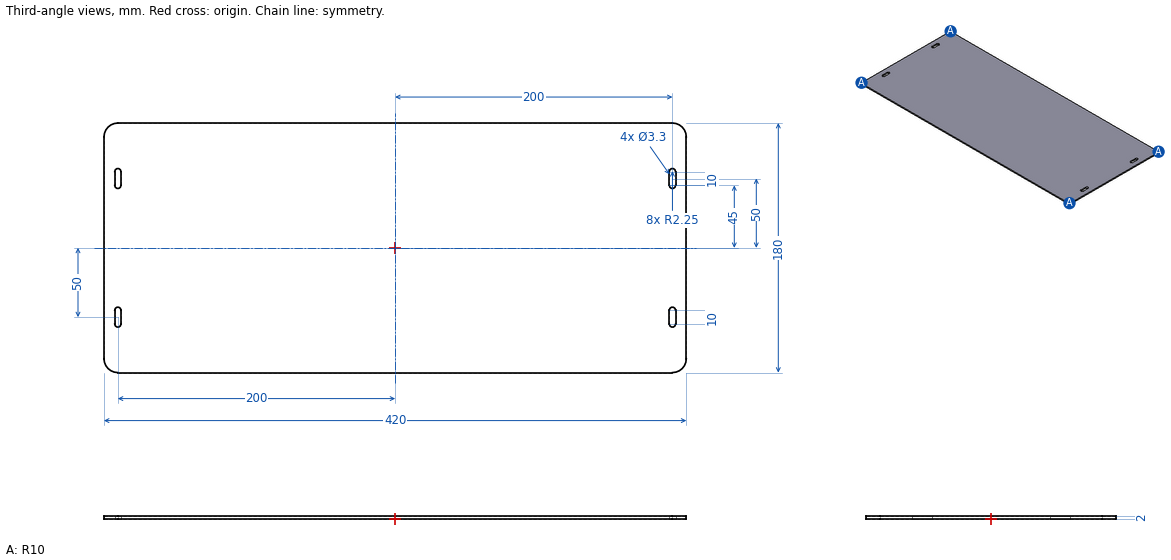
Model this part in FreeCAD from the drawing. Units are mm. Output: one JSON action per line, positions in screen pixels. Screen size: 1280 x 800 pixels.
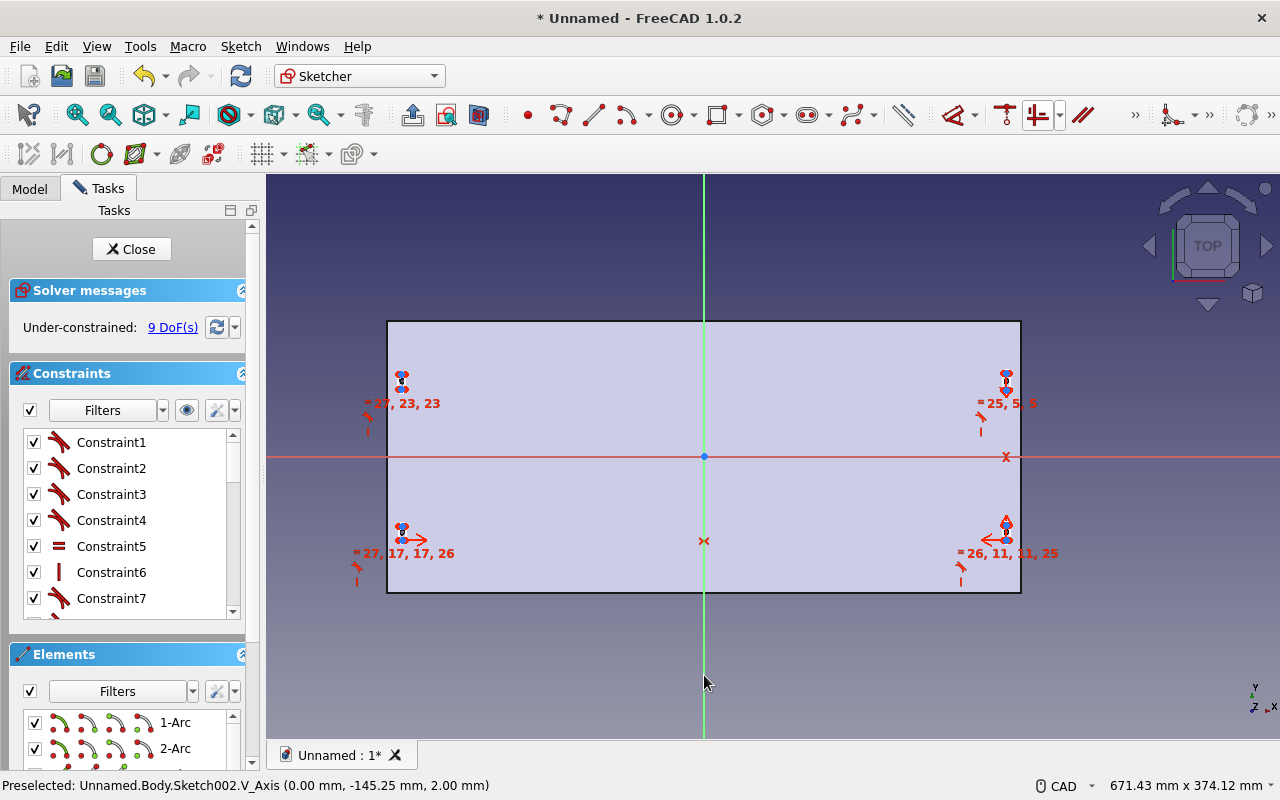
{"action": "scroll", "coordinate": [1006, 390], "scroll_direction": "up", "scroll_amount": 7}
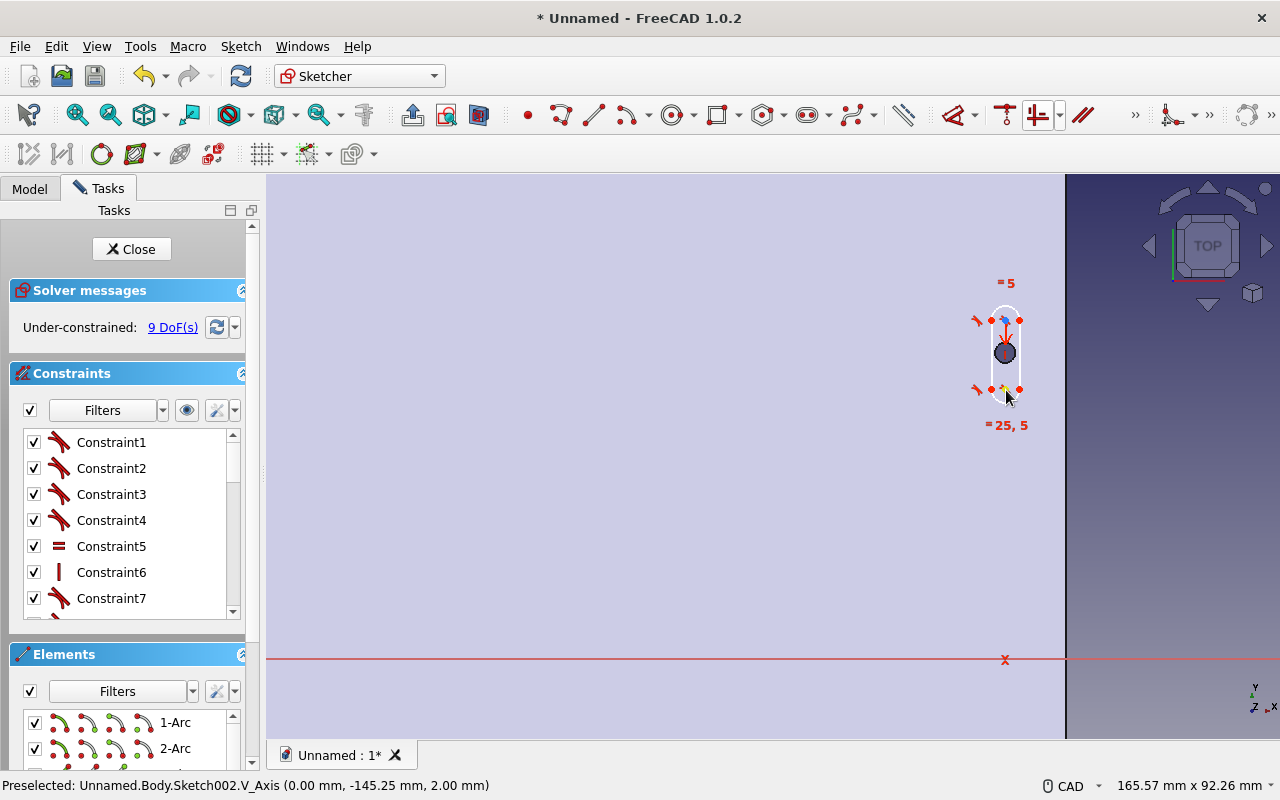
{"action": "left_click", "coordinate": [1006, 389]}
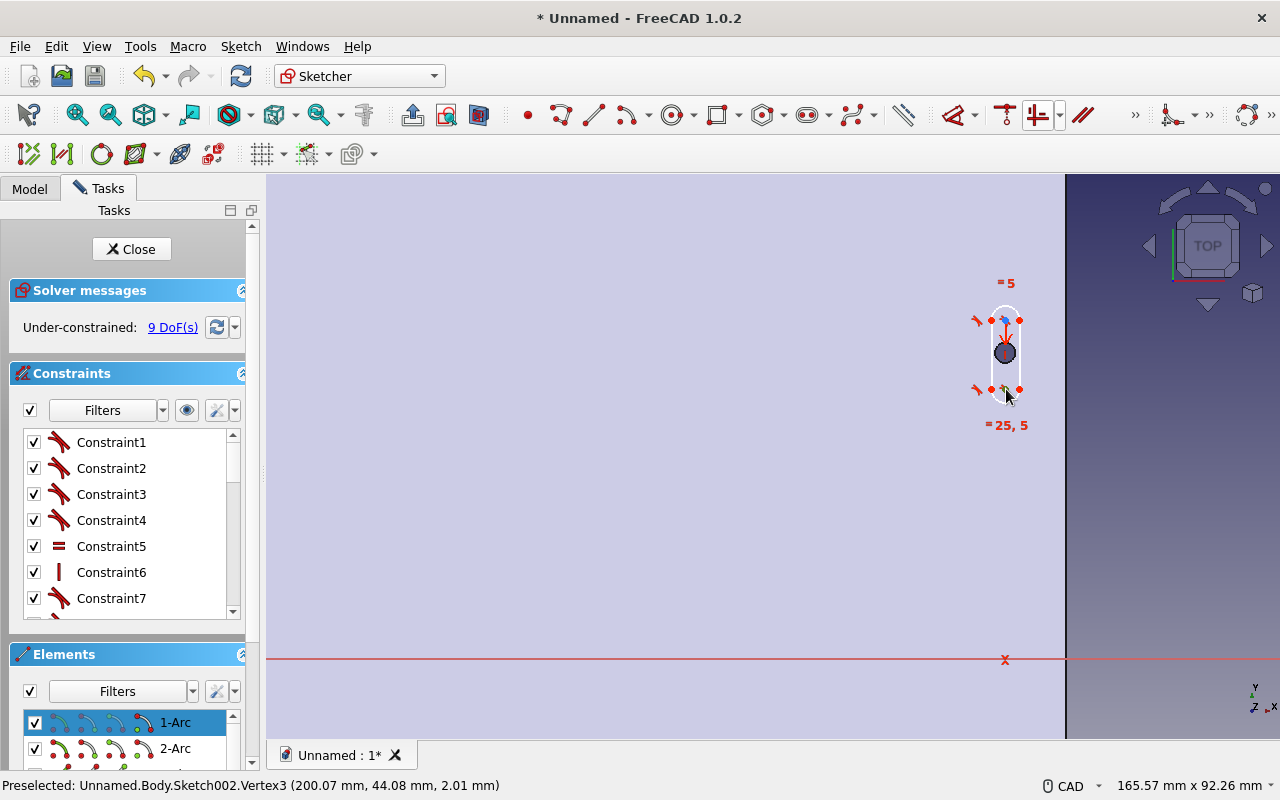
{"action": "scroll", "coordinate": [1007, 390], "scroll_direction": "down", "scroll_amount": 7}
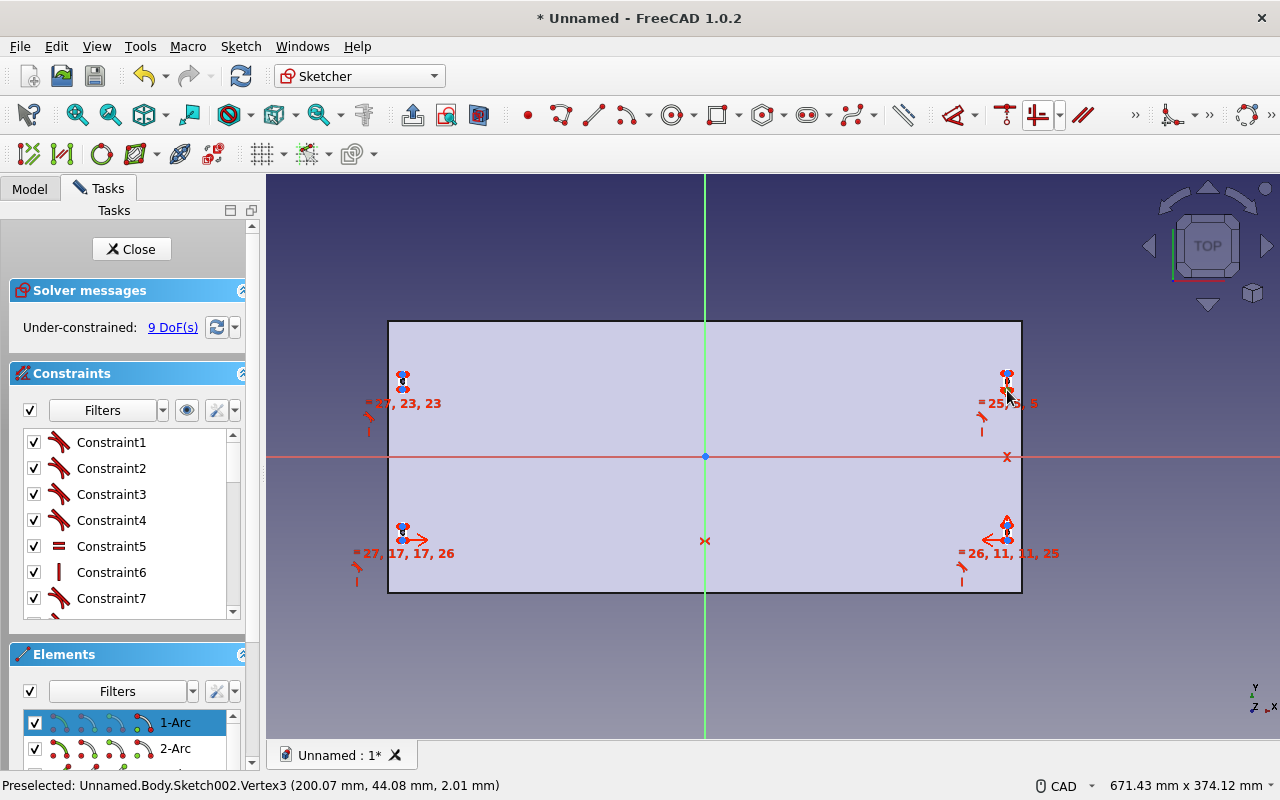
{"action": "scroll", "coordinate": [403, 390], "scroll_direction": "up", "scroll_amount": 7}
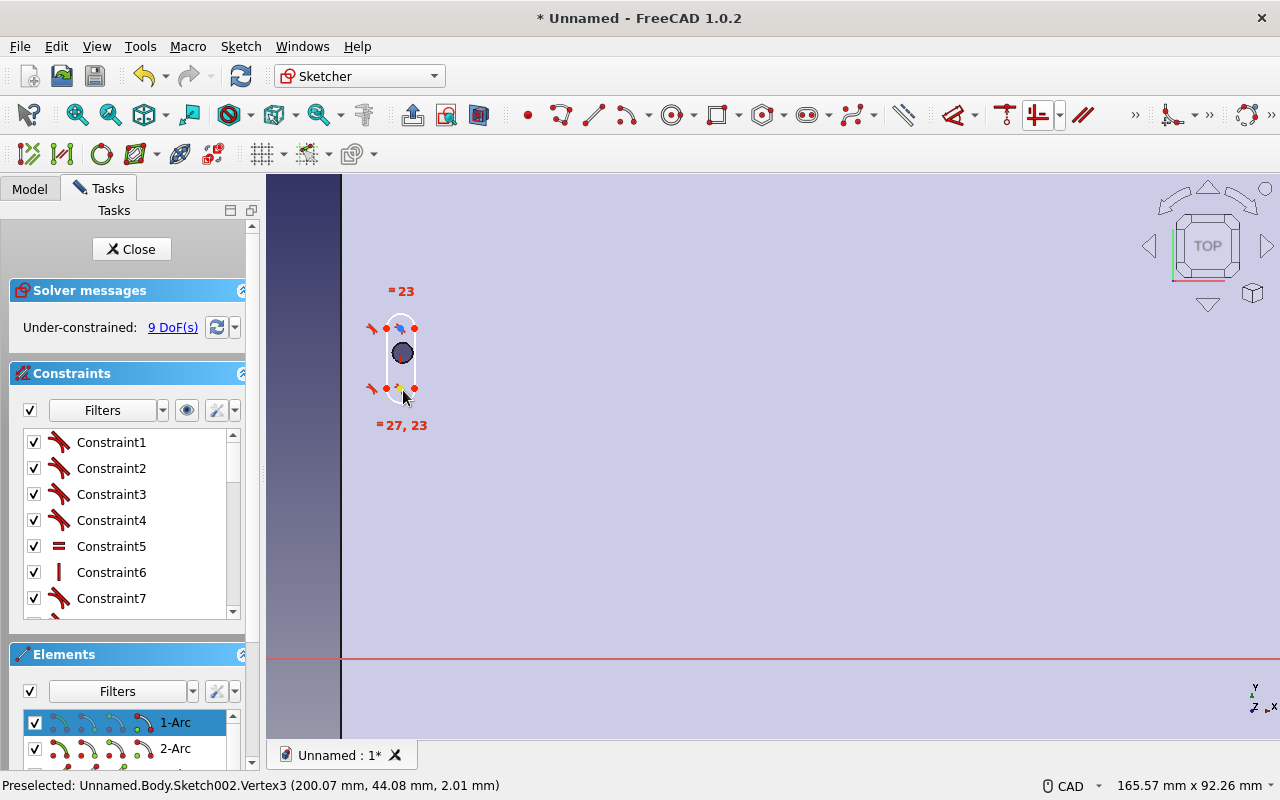
{"action": "left_click", "coordinate": [401, 389]}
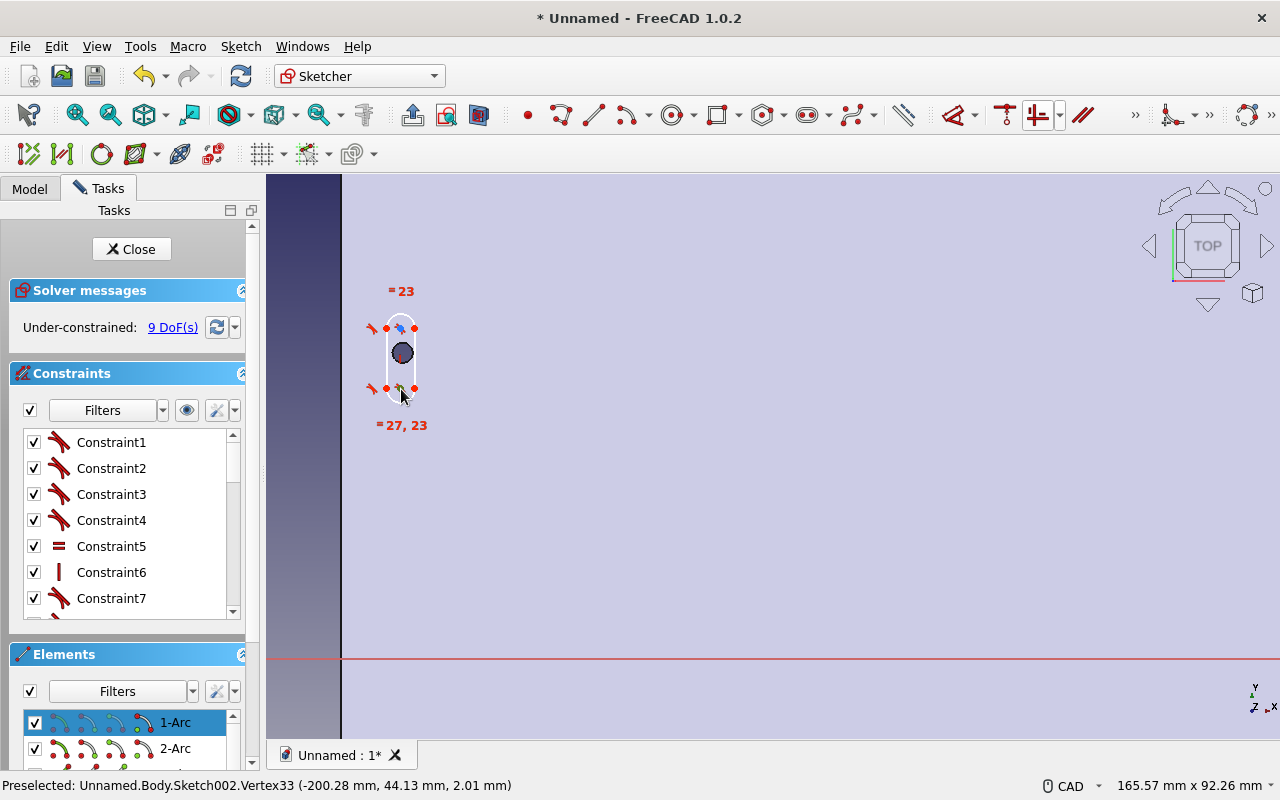
{"action": "scroll", "coordinate": [402, 390], "scroll_direction": "down", "scroll_amount": 7}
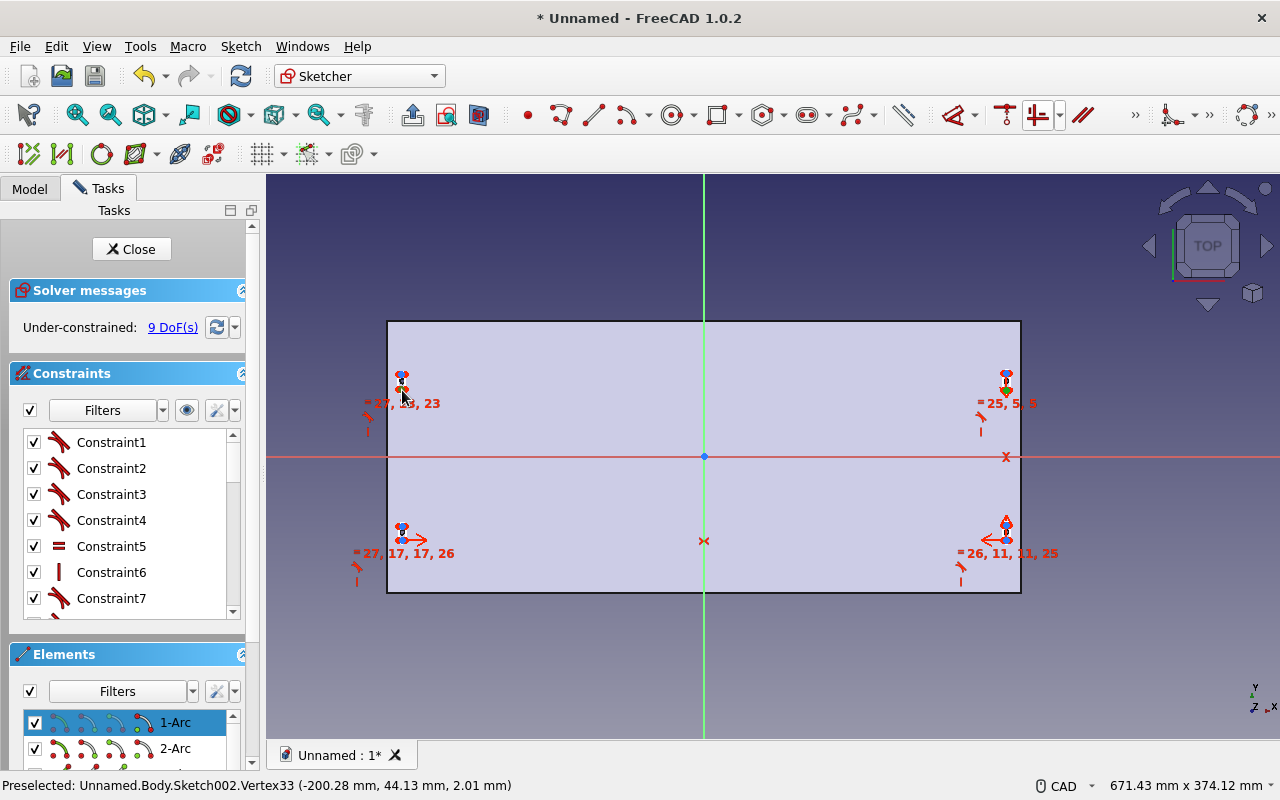
{"action": "left_click", "coordinate": [704, 675]}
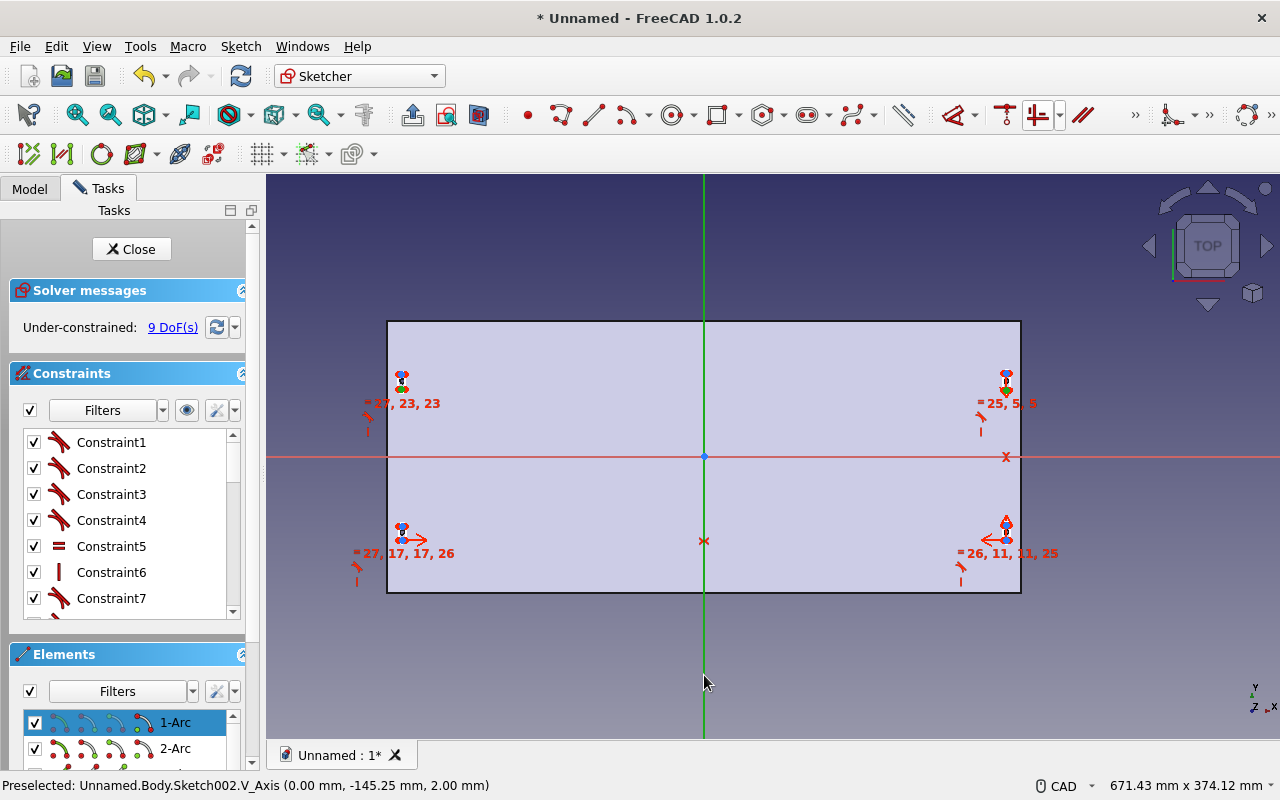
{"action": "key", "text": "s"}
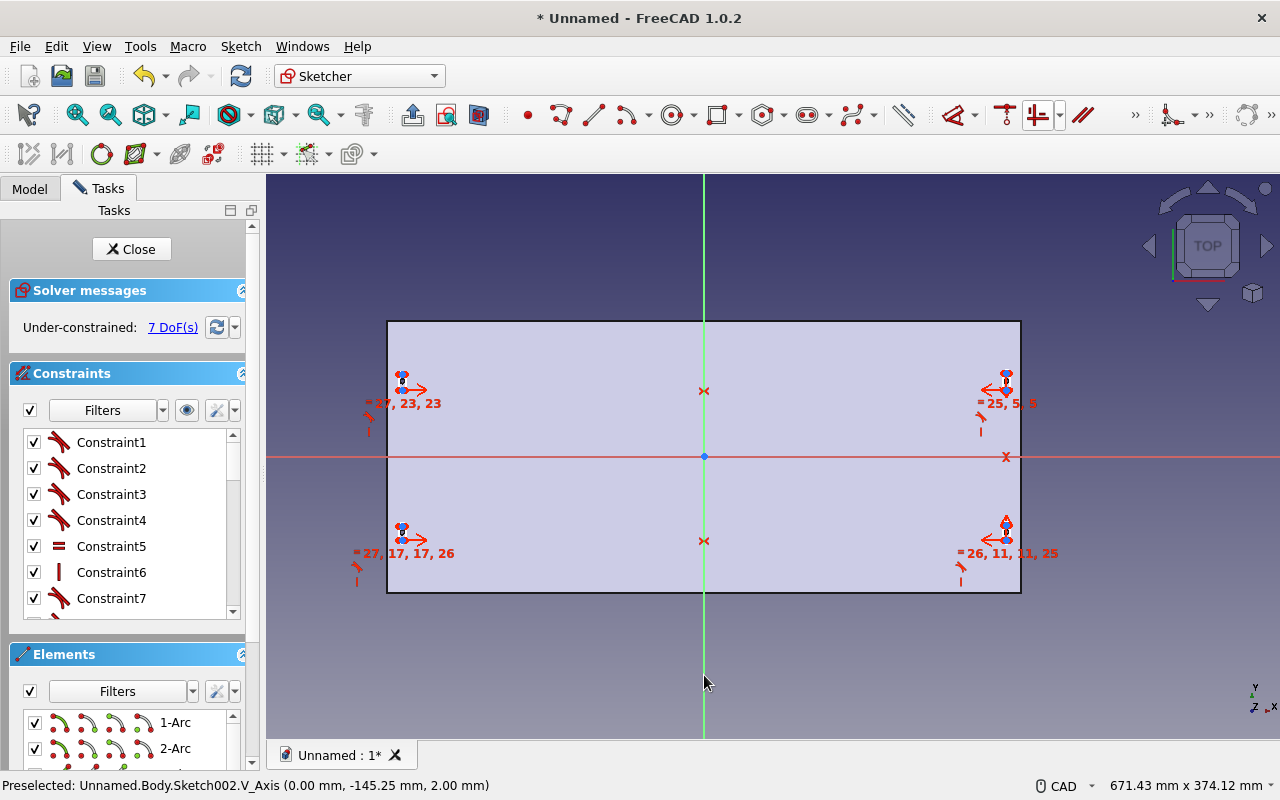
{"action": "key", "text": "d"}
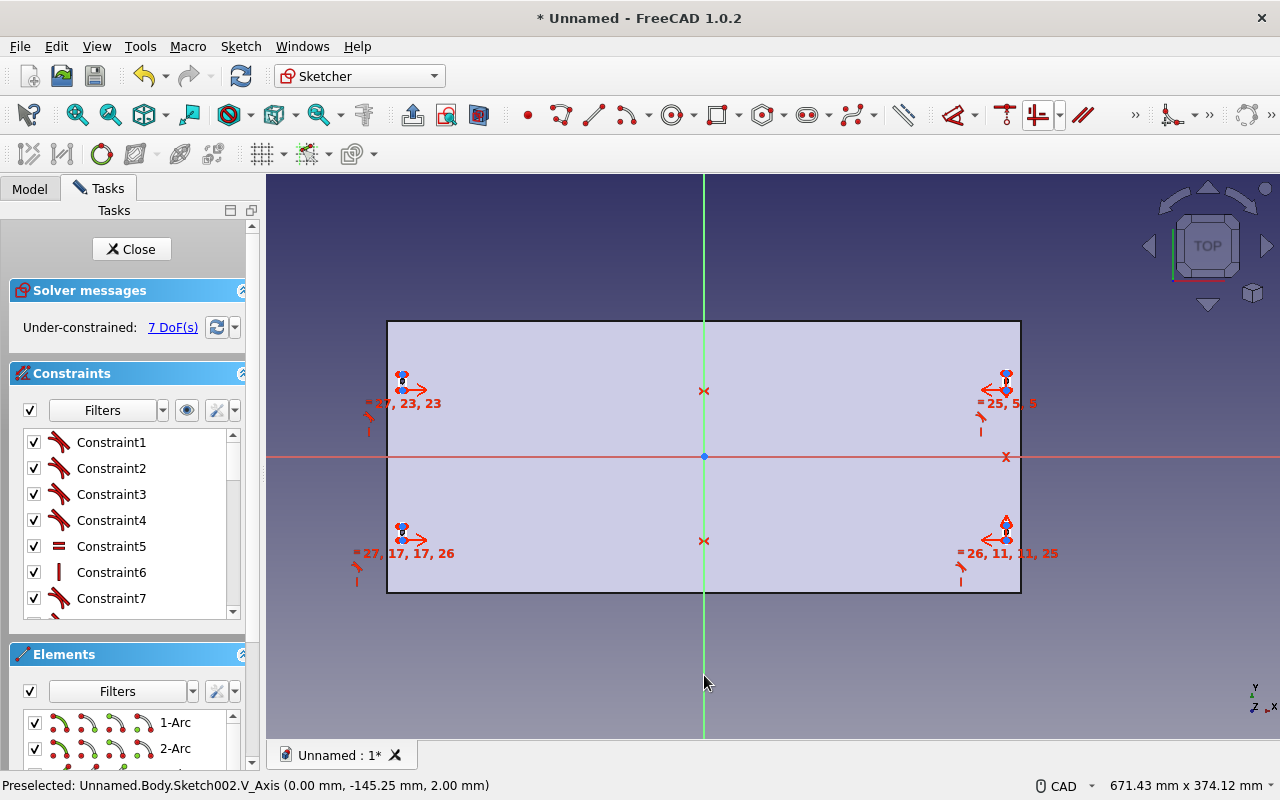
{"action": "scroll", "coordinate": [1006, 393], "scroll_direction": "up", "scroll_amount": 13}